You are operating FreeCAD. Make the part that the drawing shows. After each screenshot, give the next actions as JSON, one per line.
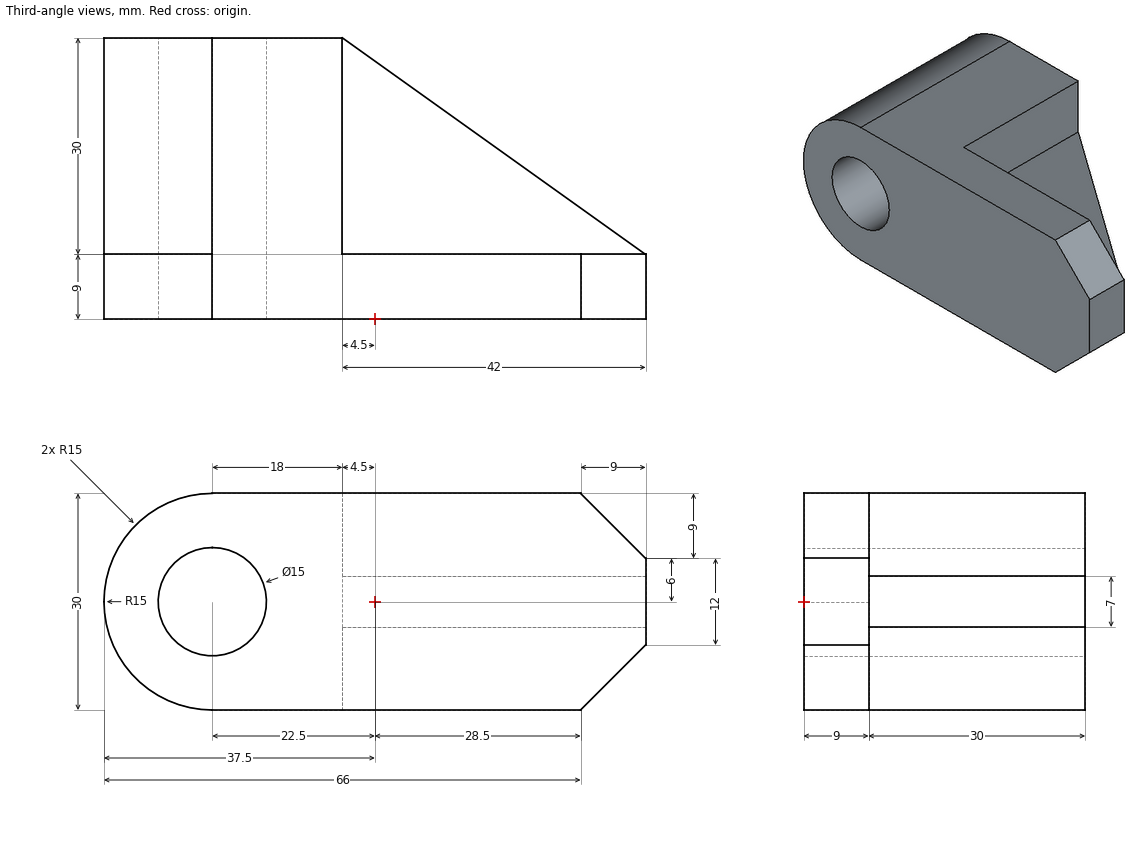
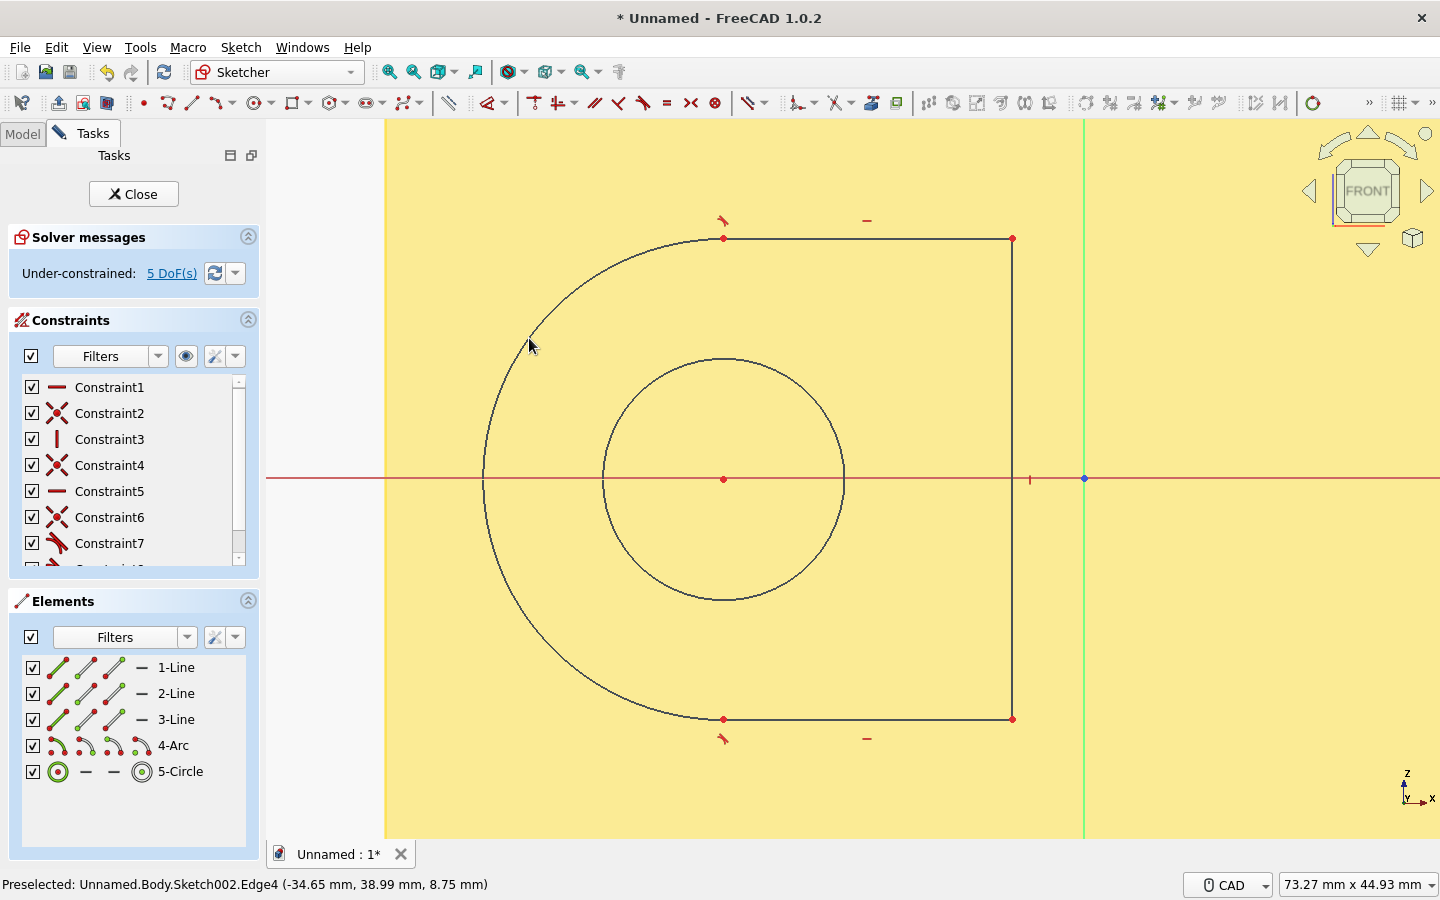
{"action": "left_click", "coordinate": [724, 480]}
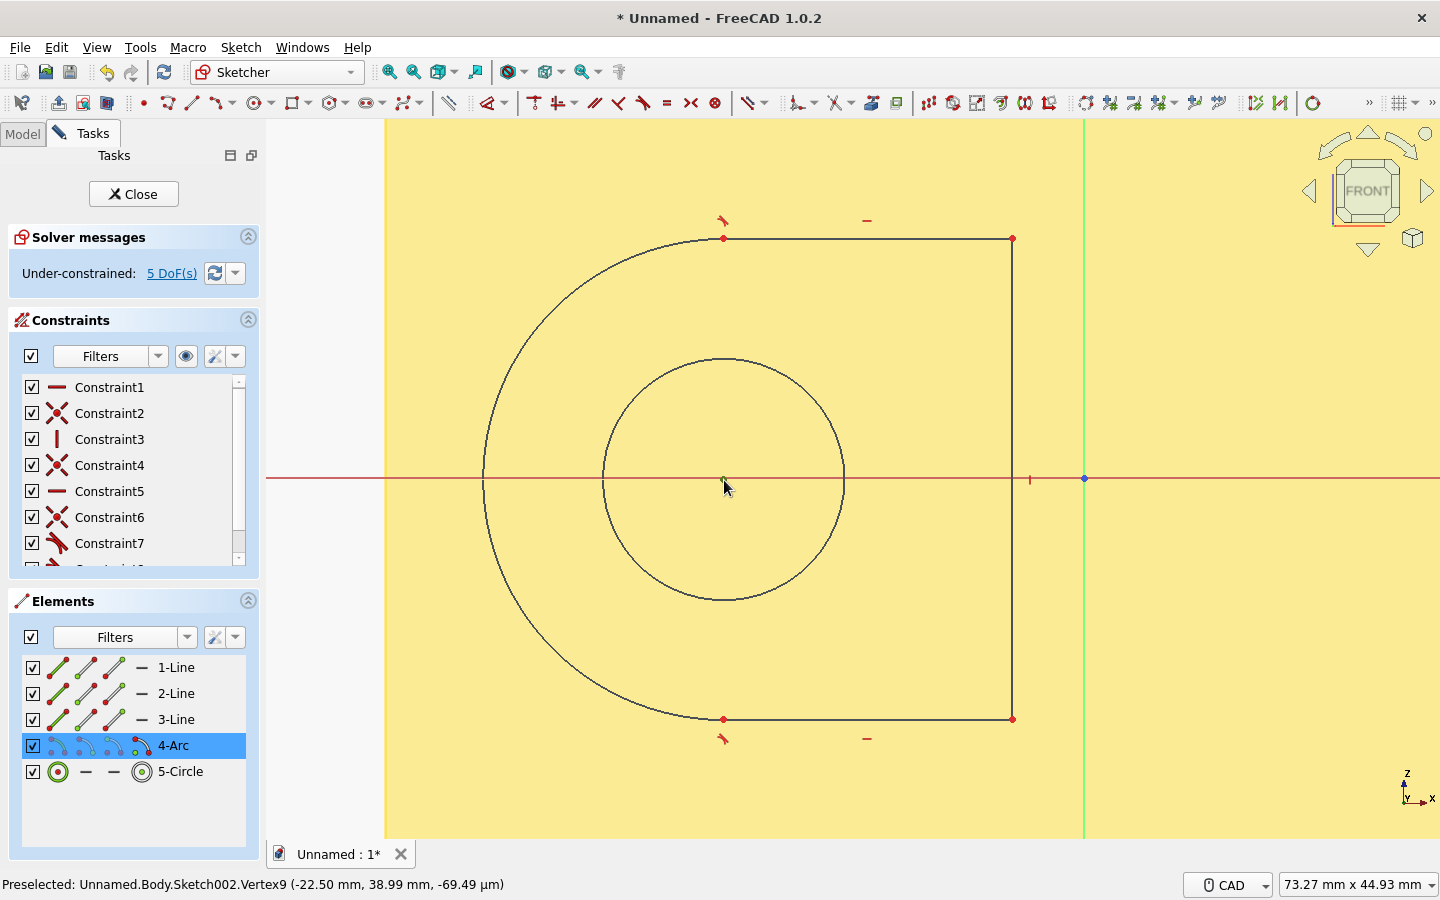
{"action": "left_click", "coordinate": [364, 478]}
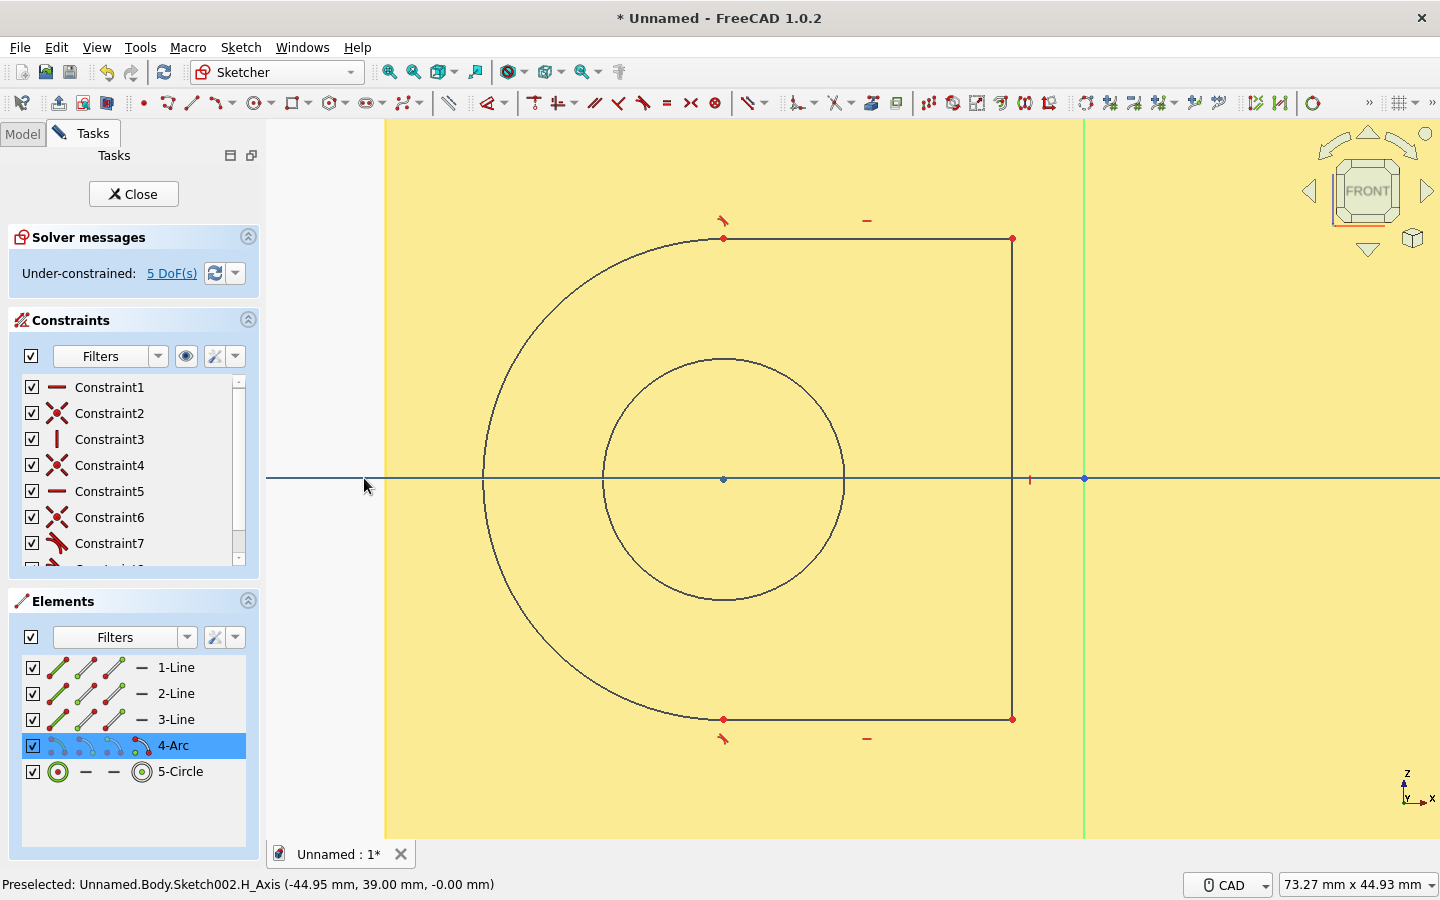
{"action": "key", "text": "c"}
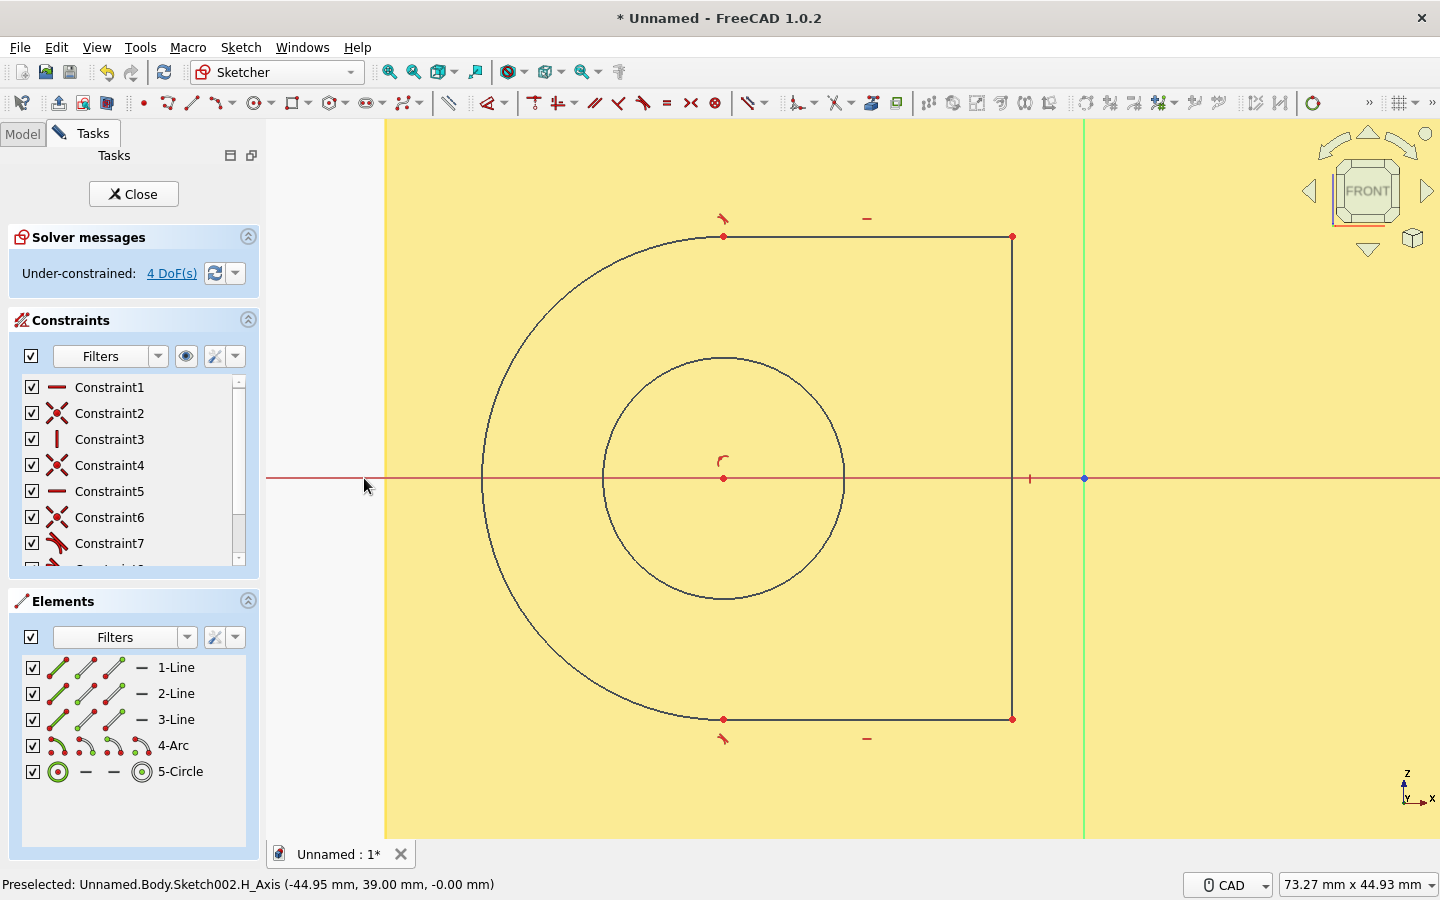
{"action": "left_click", "coordinate": [488, 104]}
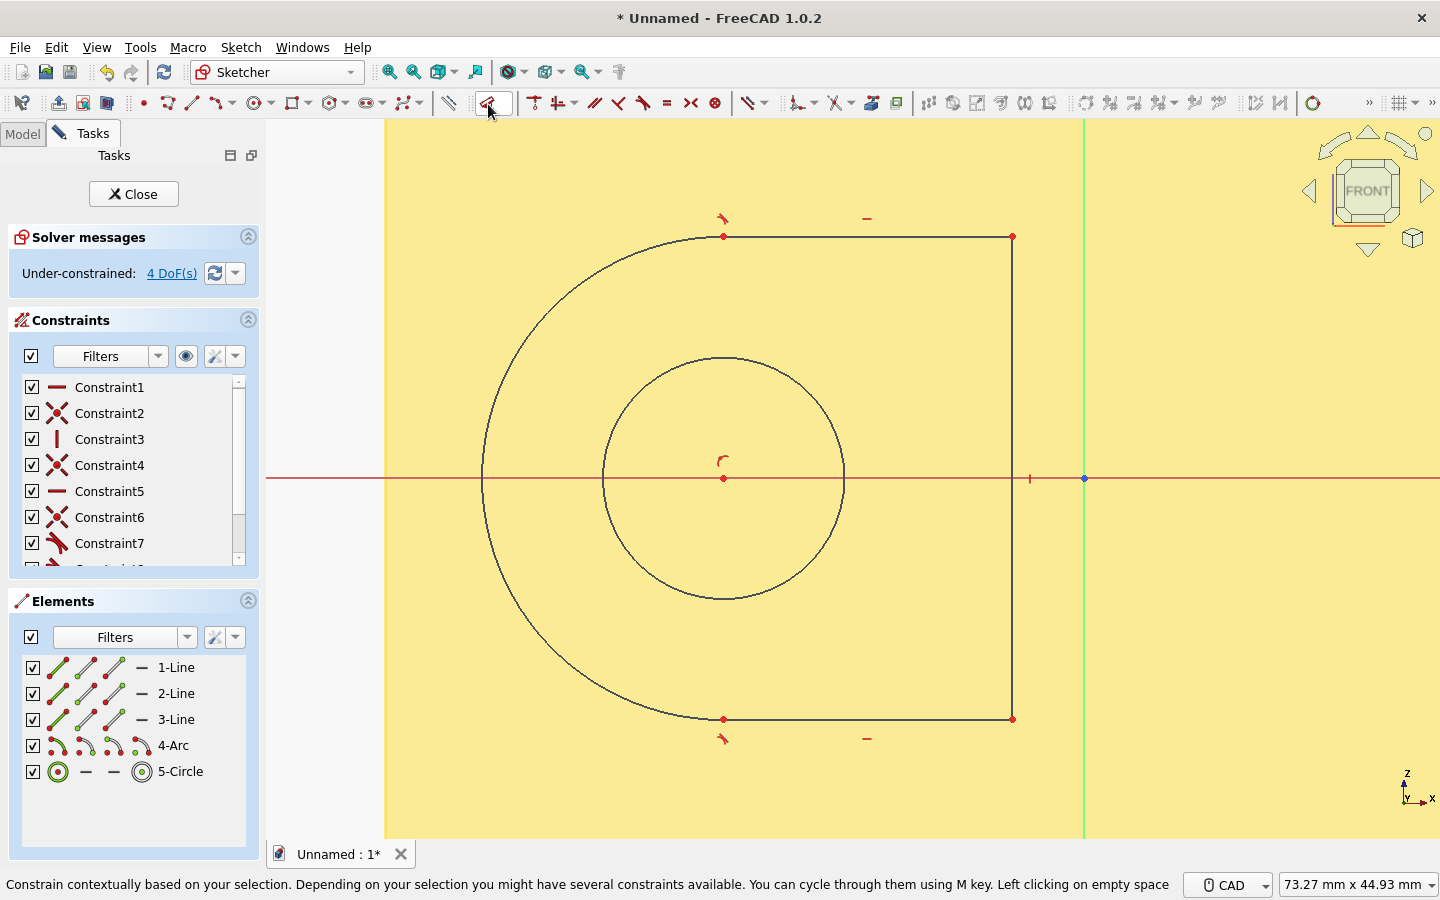
{"action": "left_click", "coordinate": [528, 336]}
{"action": "left_click", "coordinate": [502, 317]}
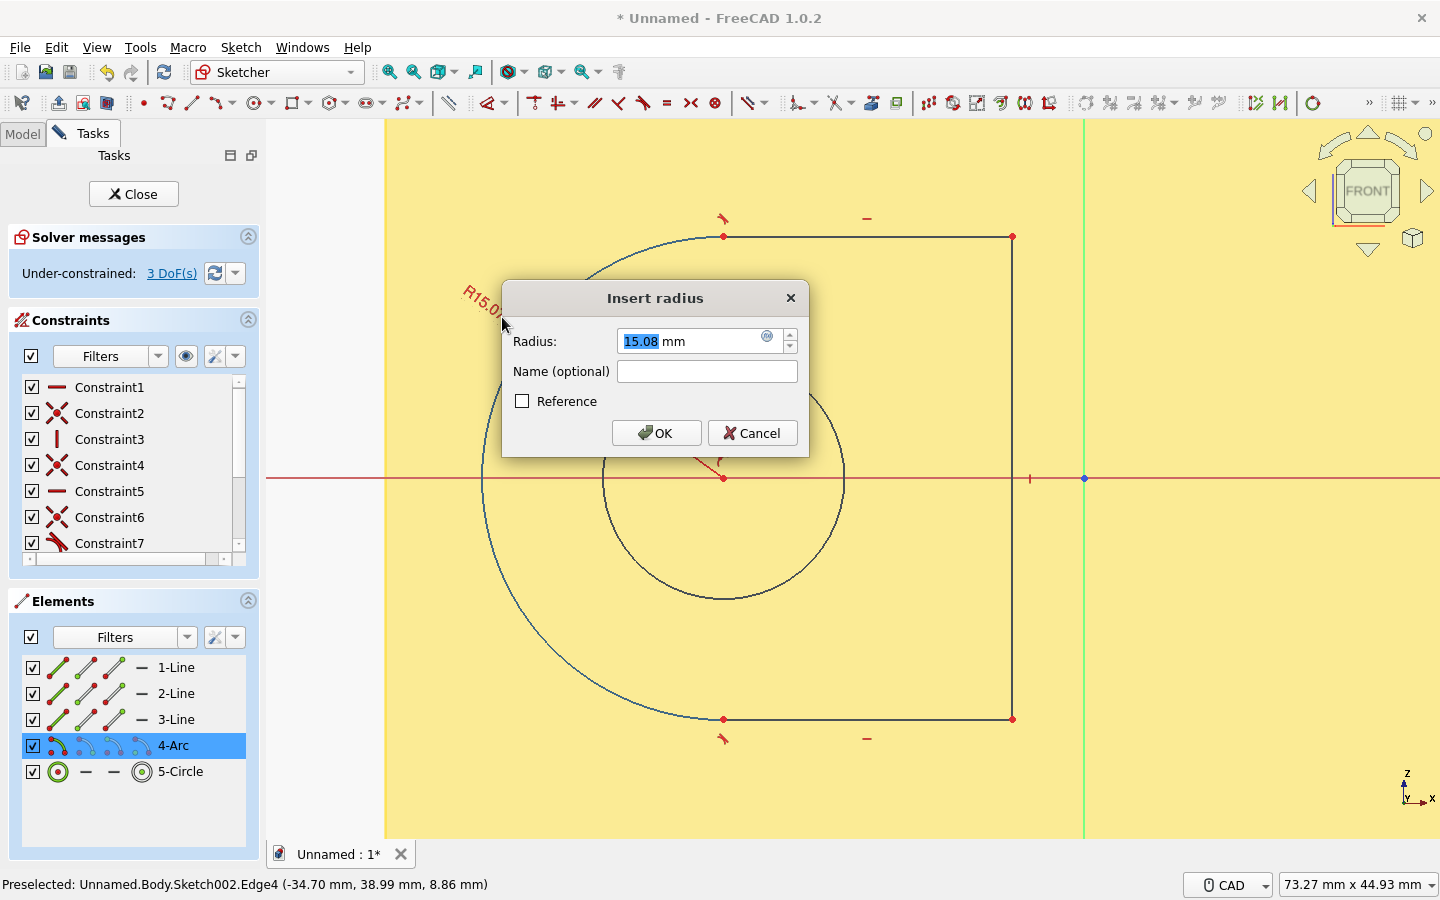
{"action": "type", "text": "15"}
{"action": "key", "text": "Return"}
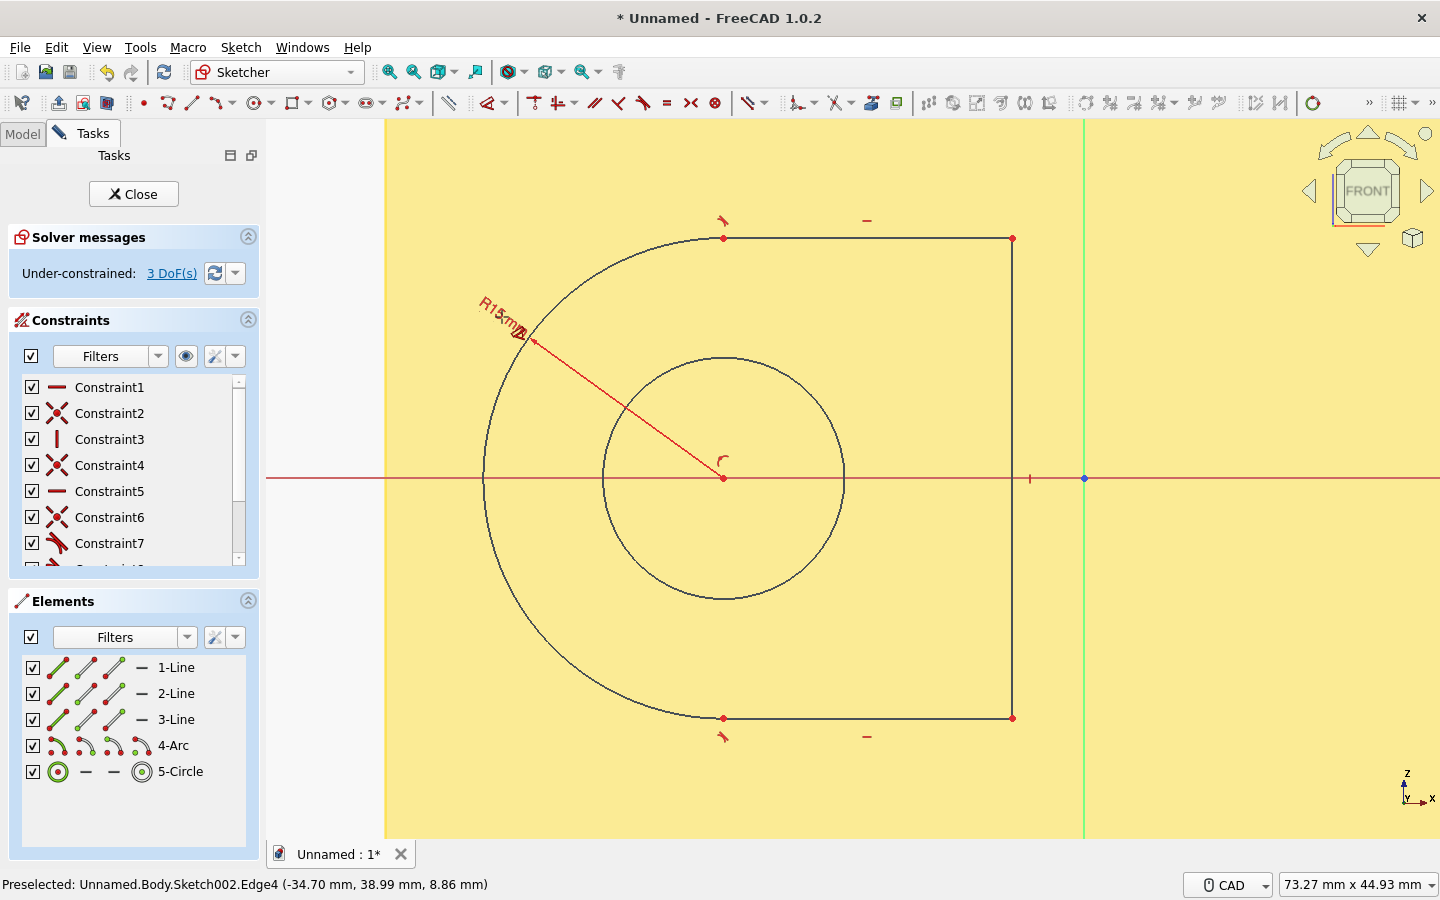
{"action": "left_click", "coordinate": [809, 393]}
{"action": "left_click", "coordinate": [832, 370]}